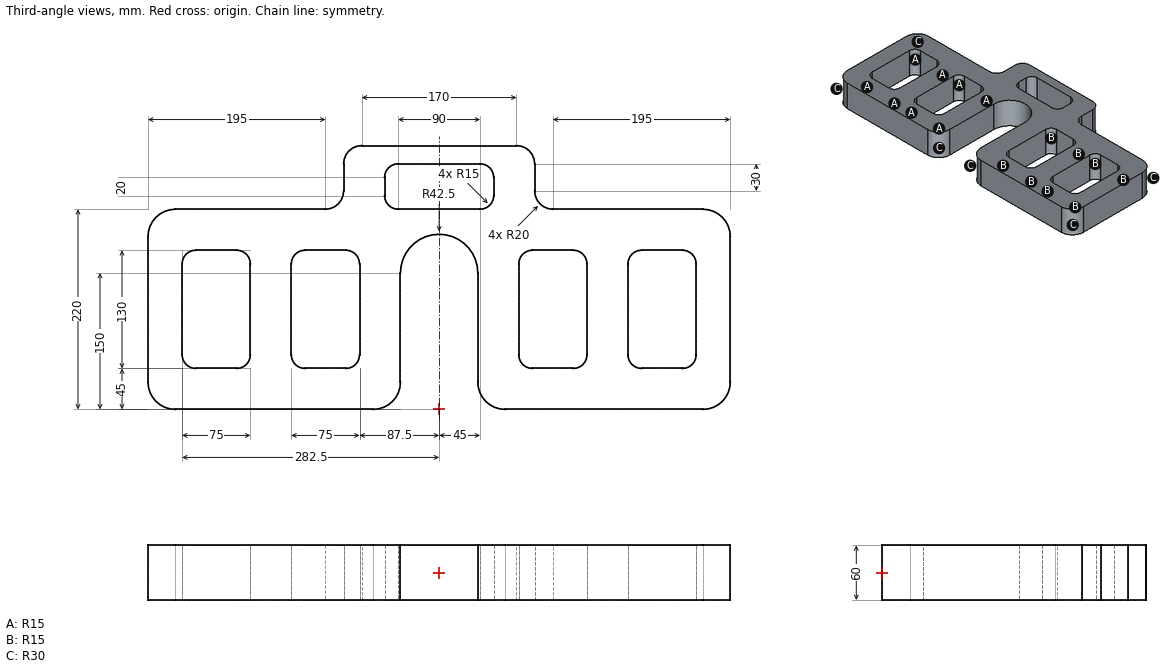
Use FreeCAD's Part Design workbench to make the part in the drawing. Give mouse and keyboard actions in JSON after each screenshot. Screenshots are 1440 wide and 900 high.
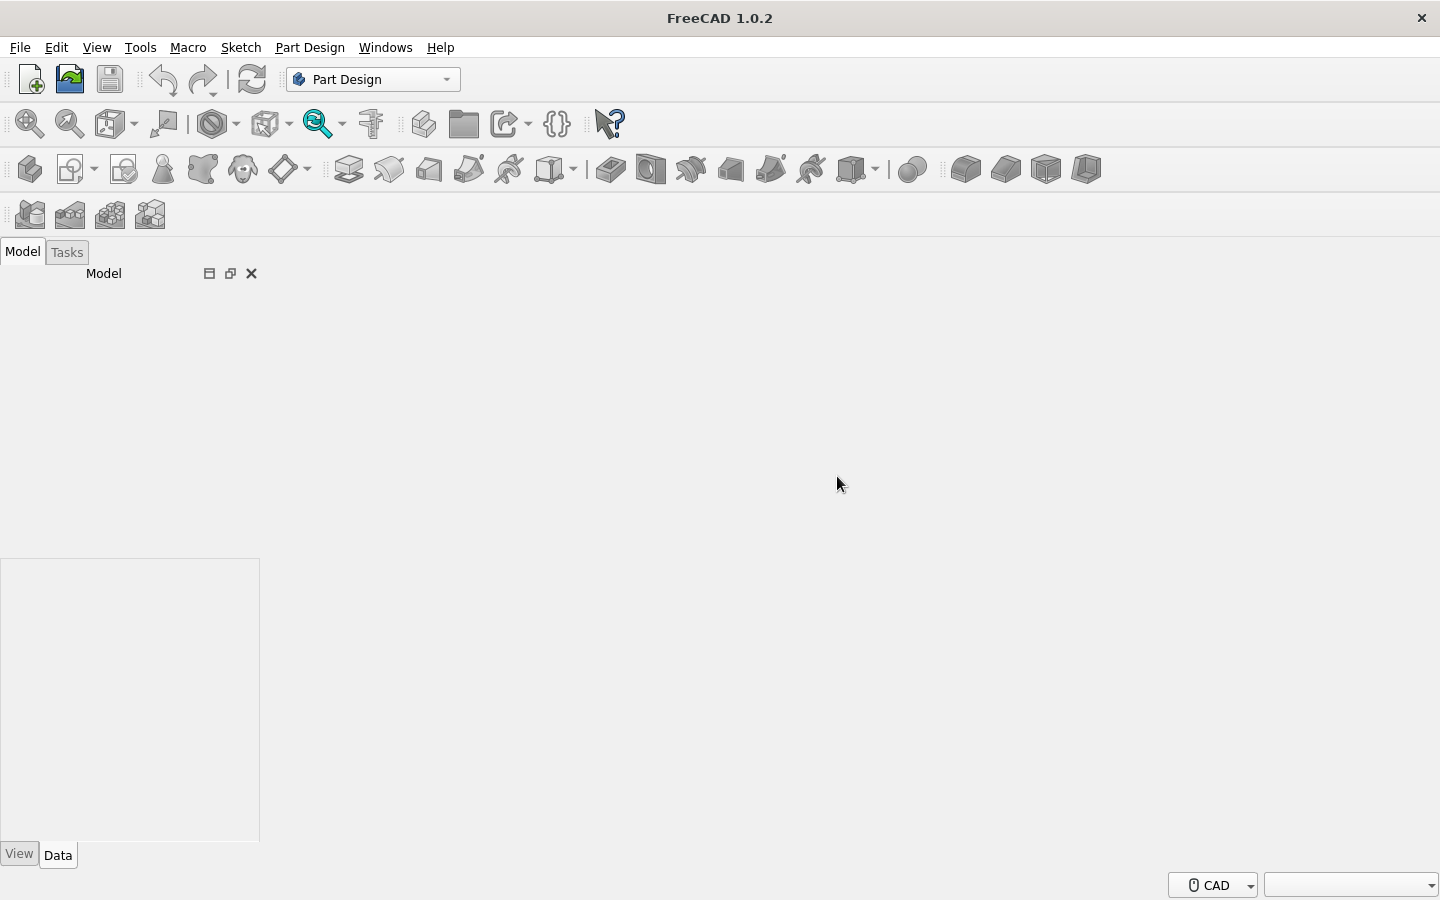
{"action": "key", "text": "ctrl+n"}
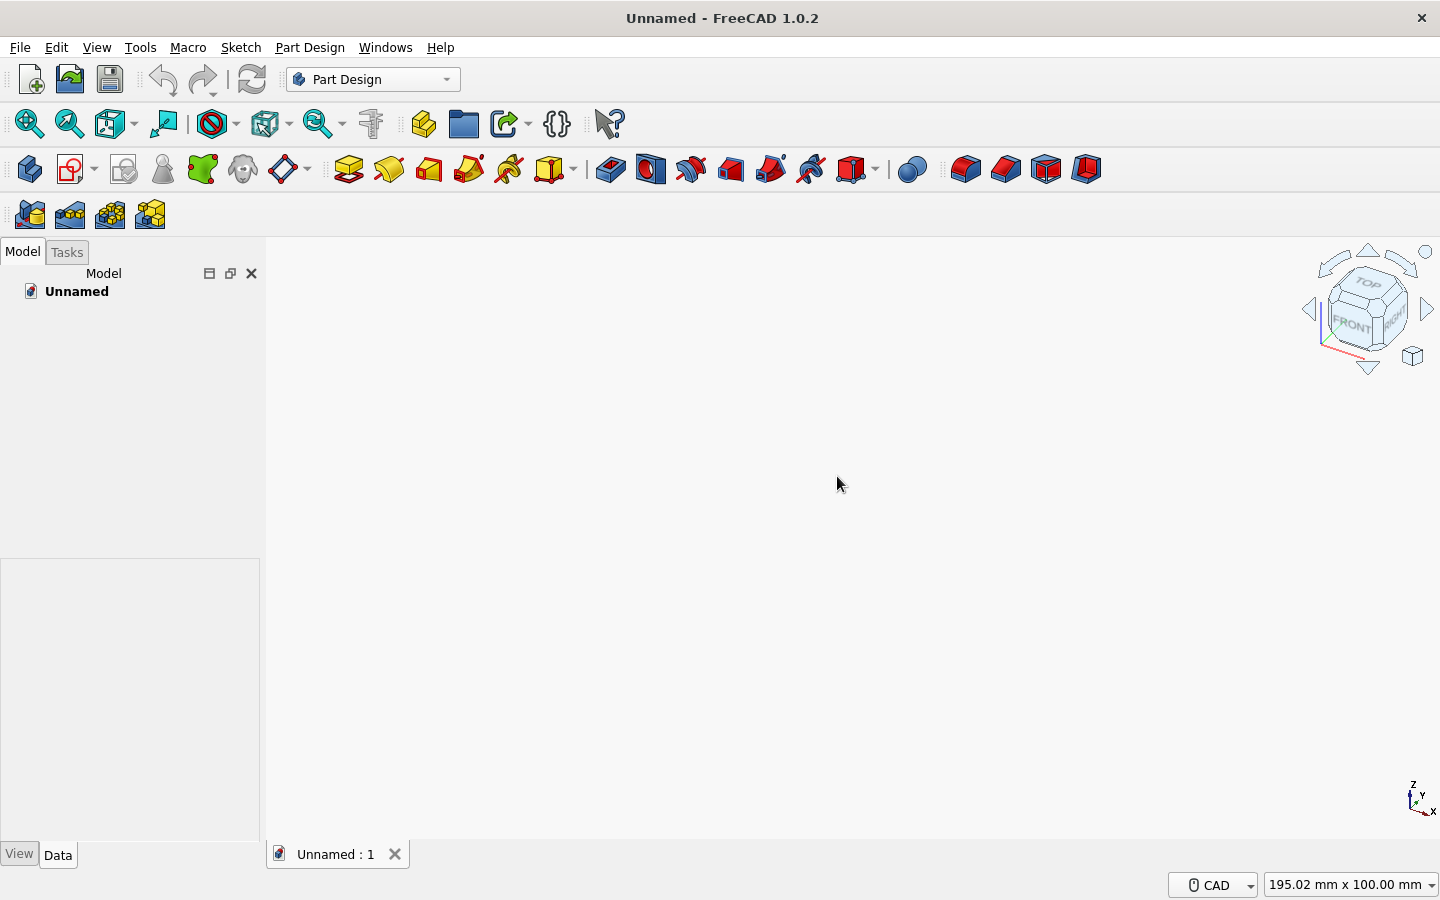
{"action": "left_click", "coordinate": [70, 170]}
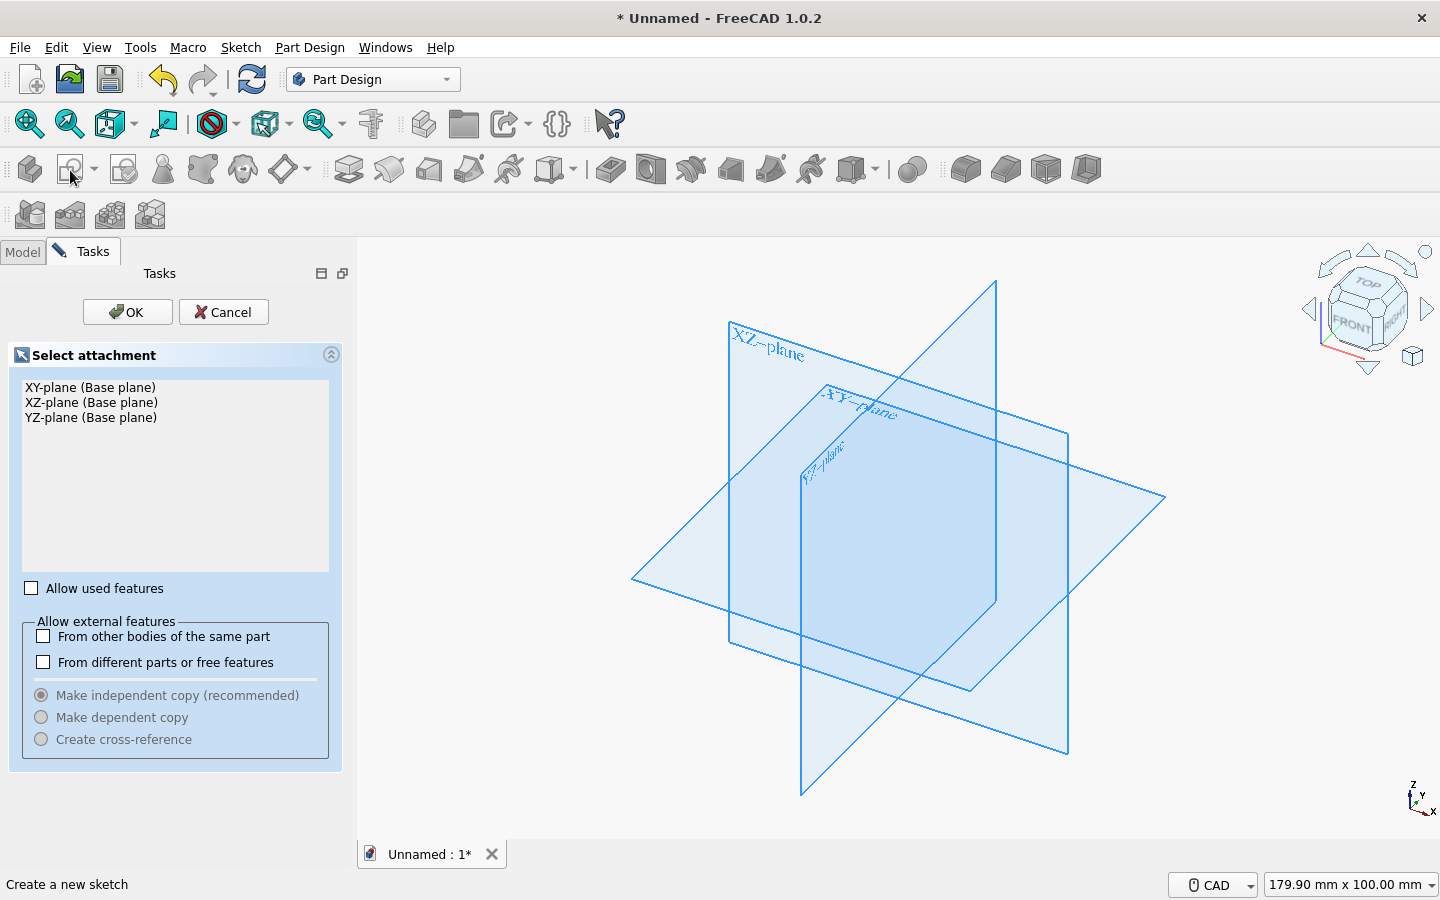
{"action": "left_click", "coordinate": [82, 388]}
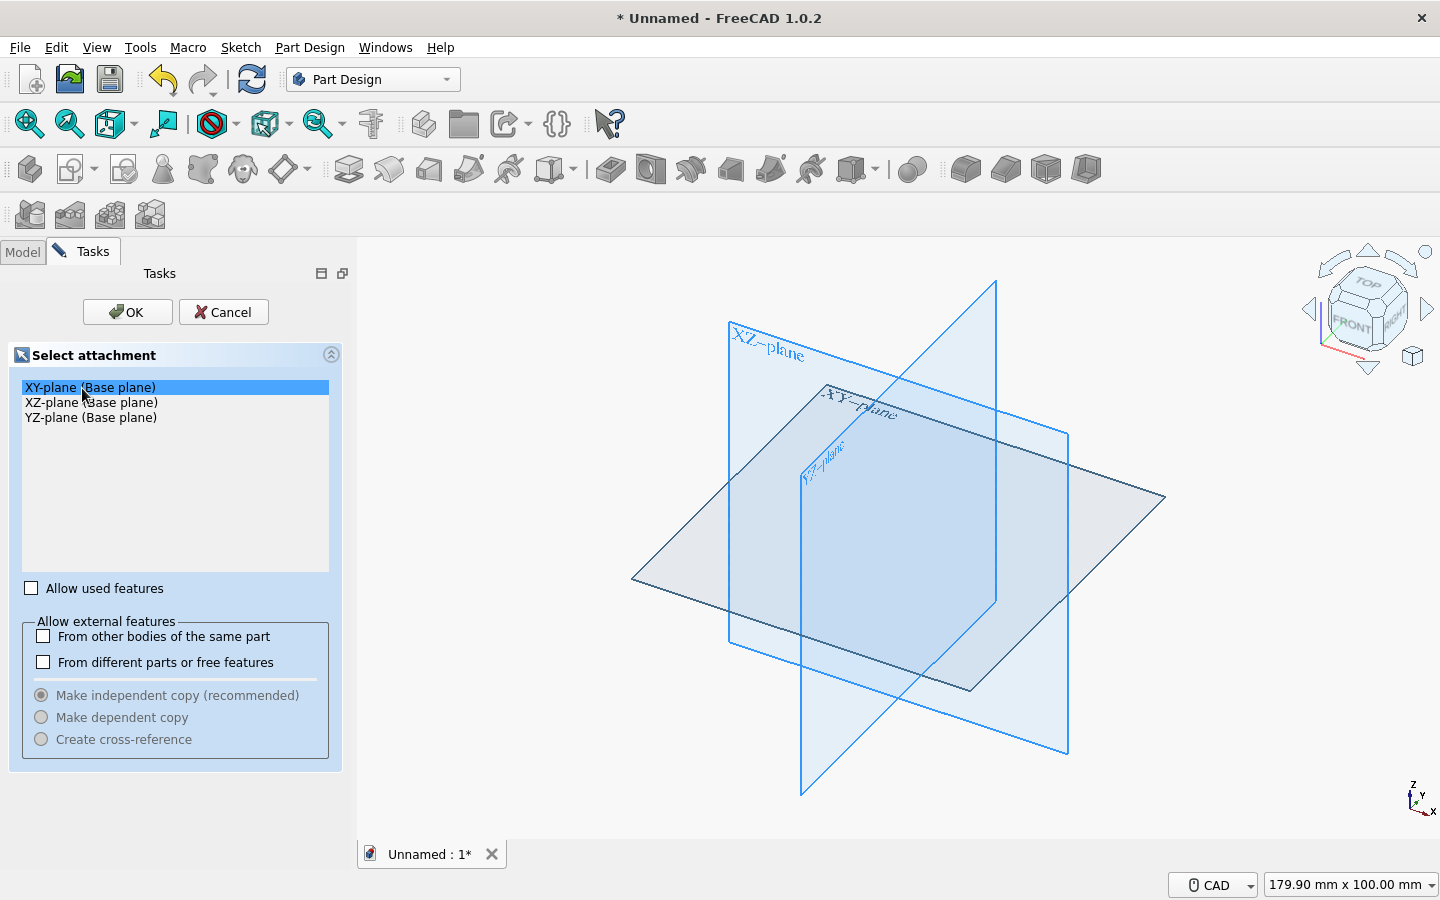
{"action": "left_click", "coordinate": [128, 312]}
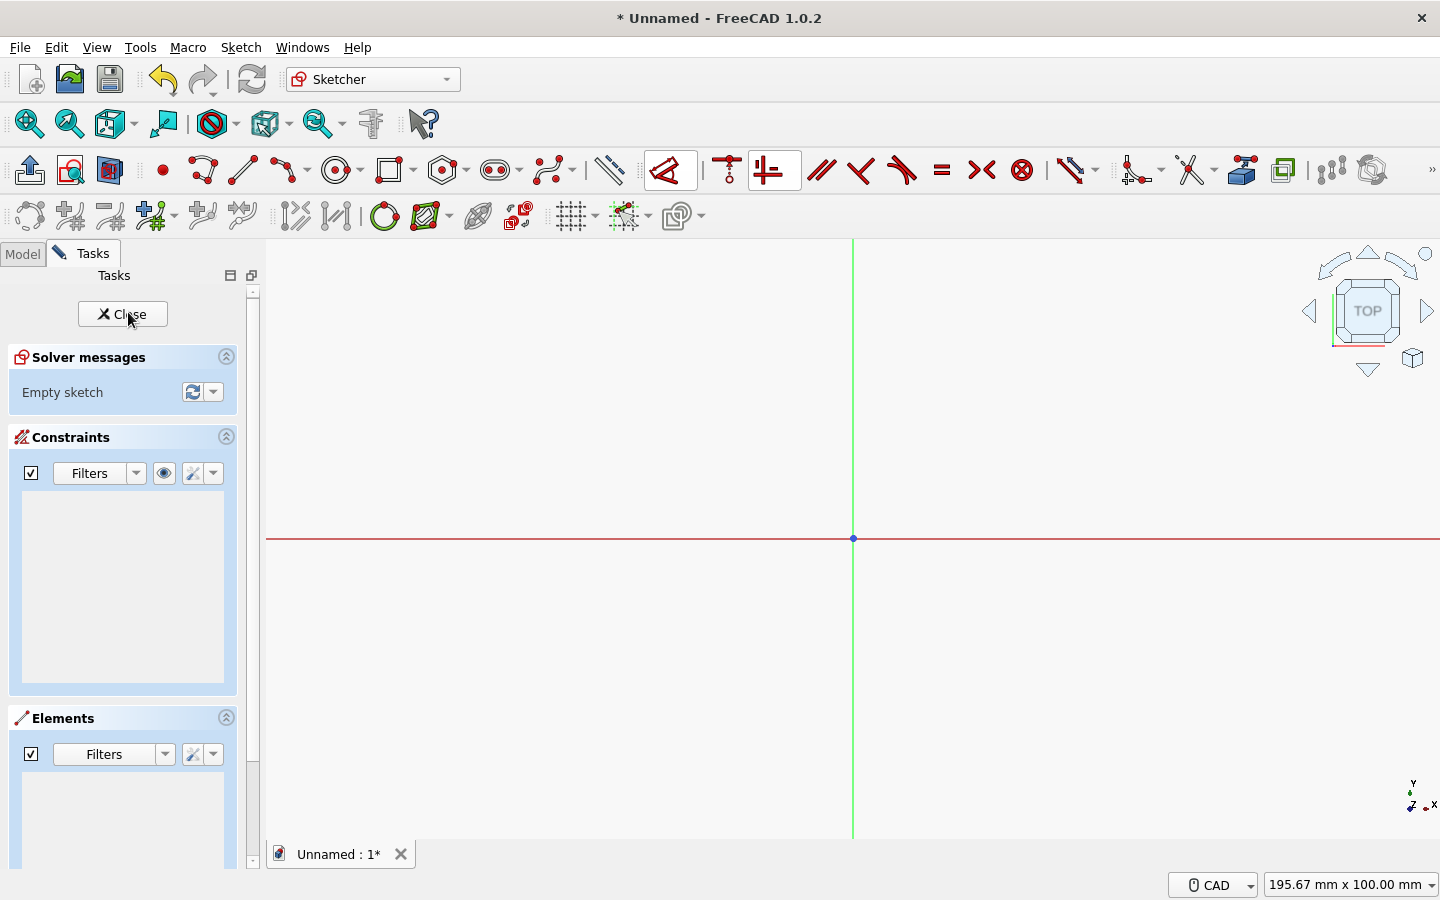
{"action": "scroll", "coordinate": [771, 711], "scroll_direction": "down", "scroll_amount": 9}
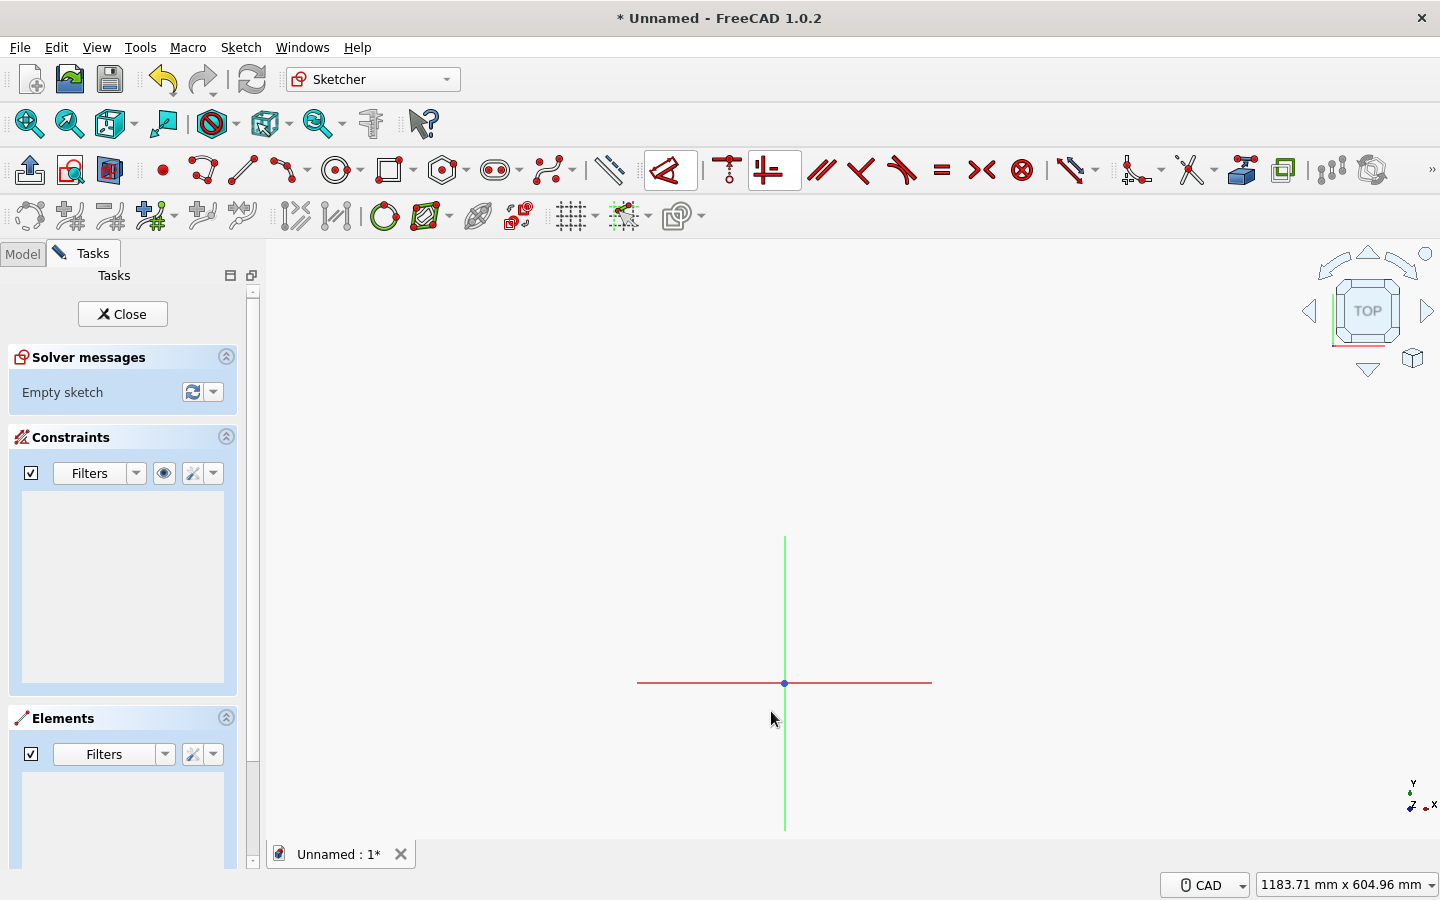
{"action": "left_click", "coordinate": [244, 170]}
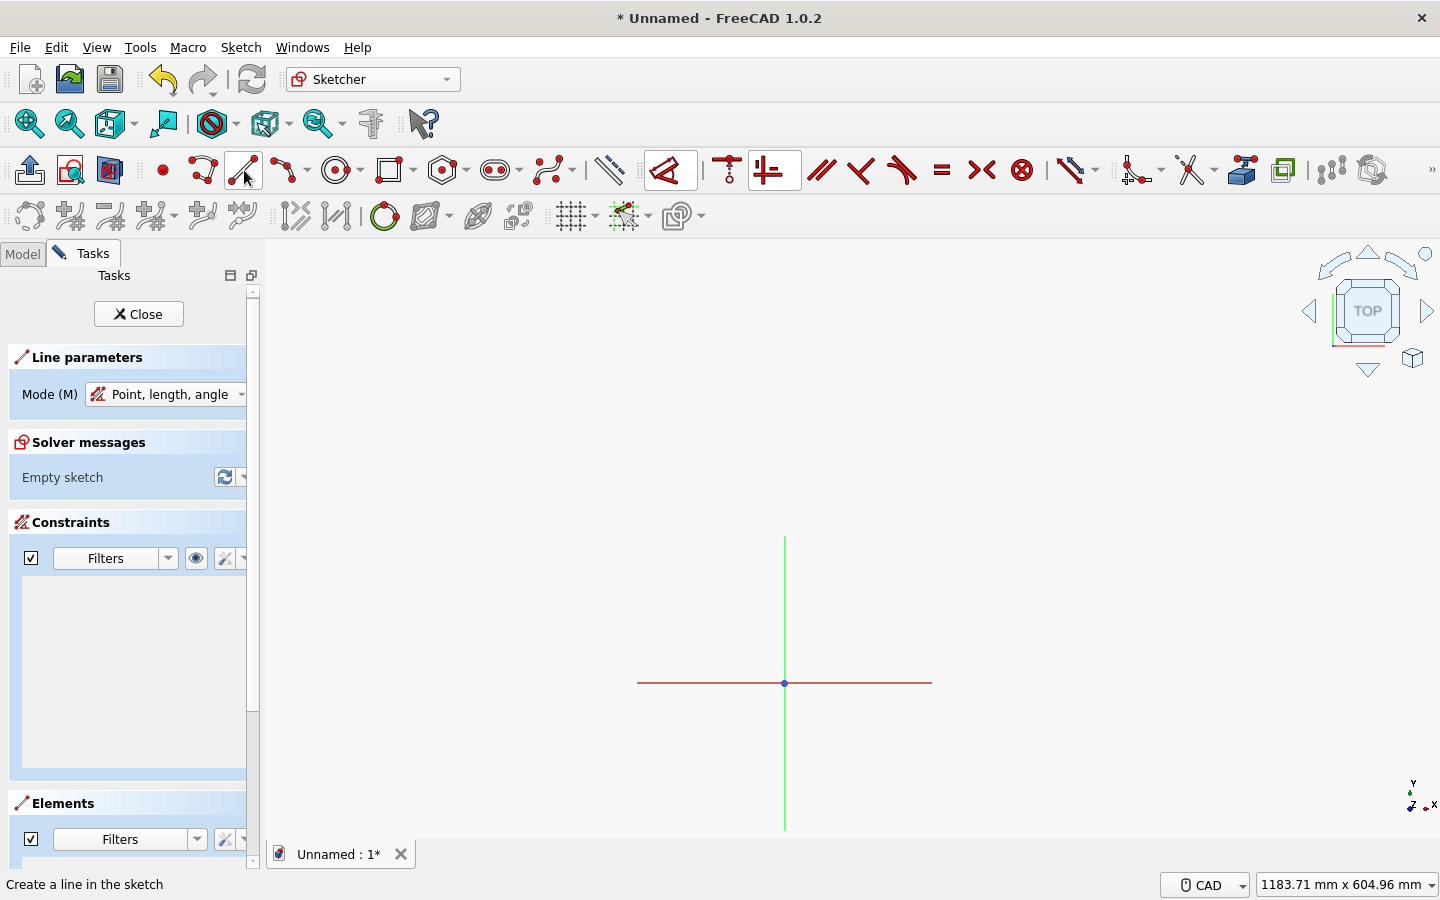
{"action": "left_click", "coordinate": [889, 445]}
{"action": "left_click", "coordinate": [889, 415]}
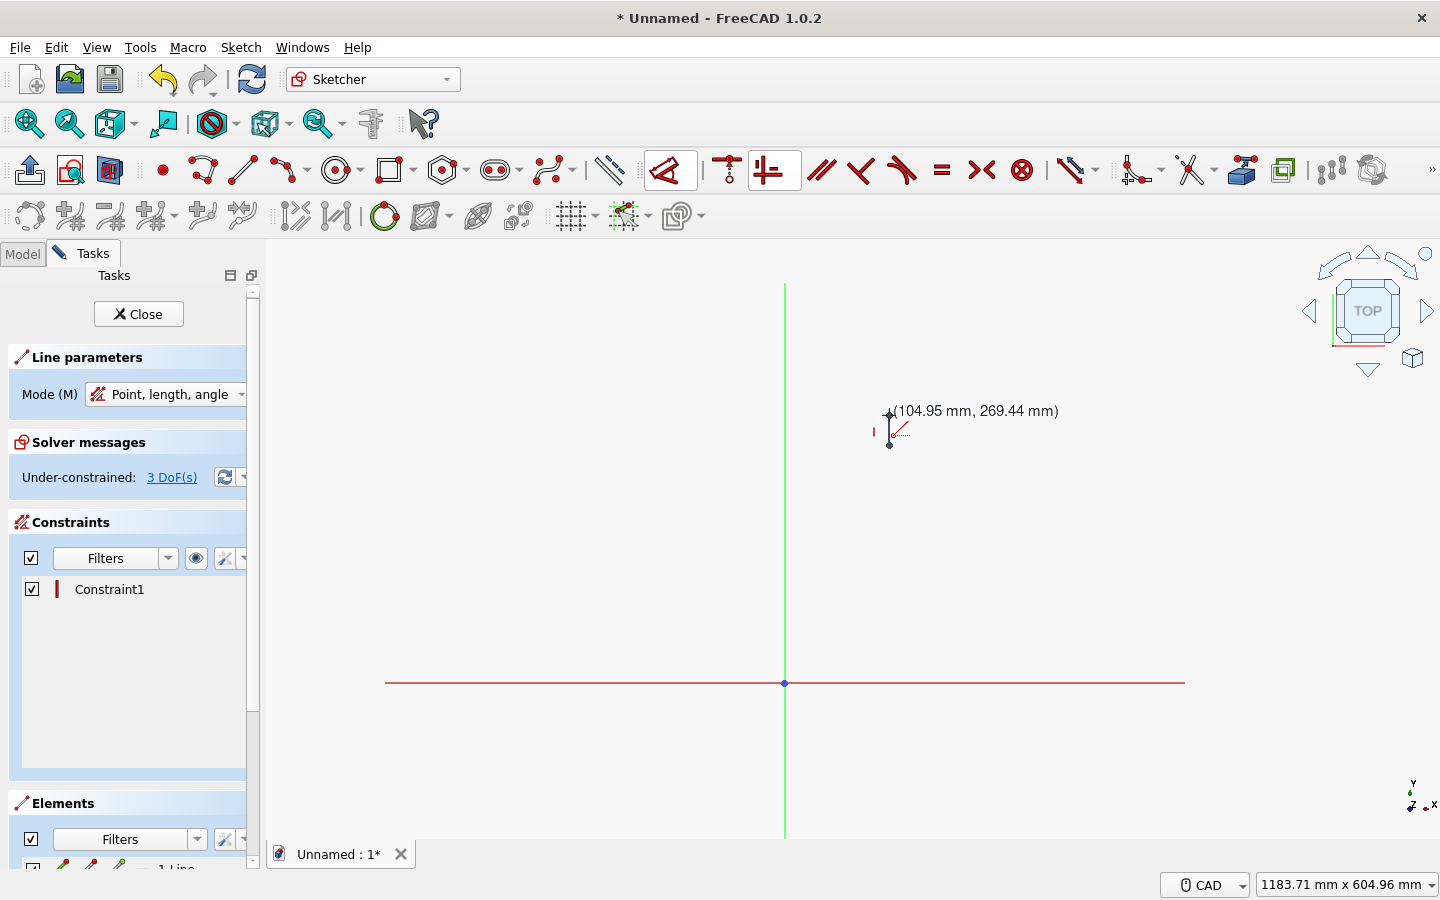
{"action": "left_click", "coordinate": [869, 396]}
{"action": "left_click", "coordinate": [701, 396]}